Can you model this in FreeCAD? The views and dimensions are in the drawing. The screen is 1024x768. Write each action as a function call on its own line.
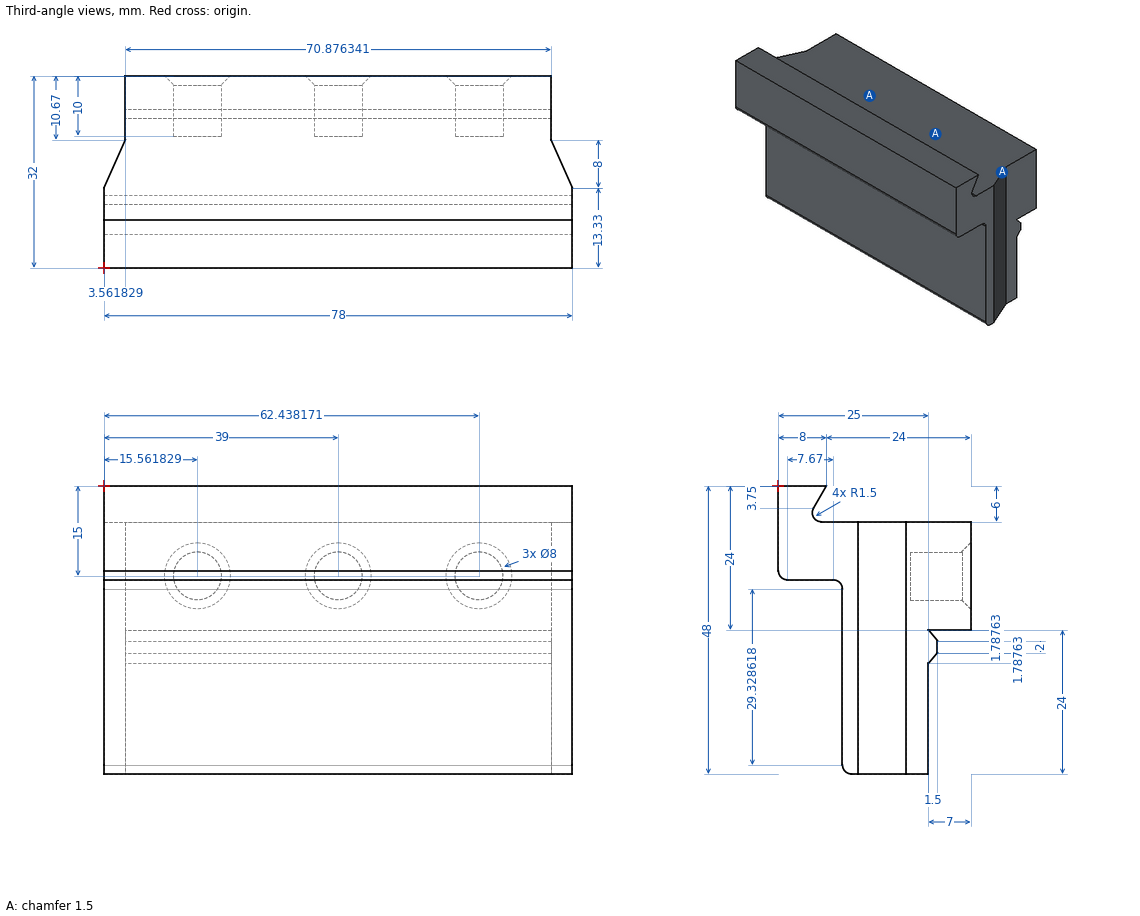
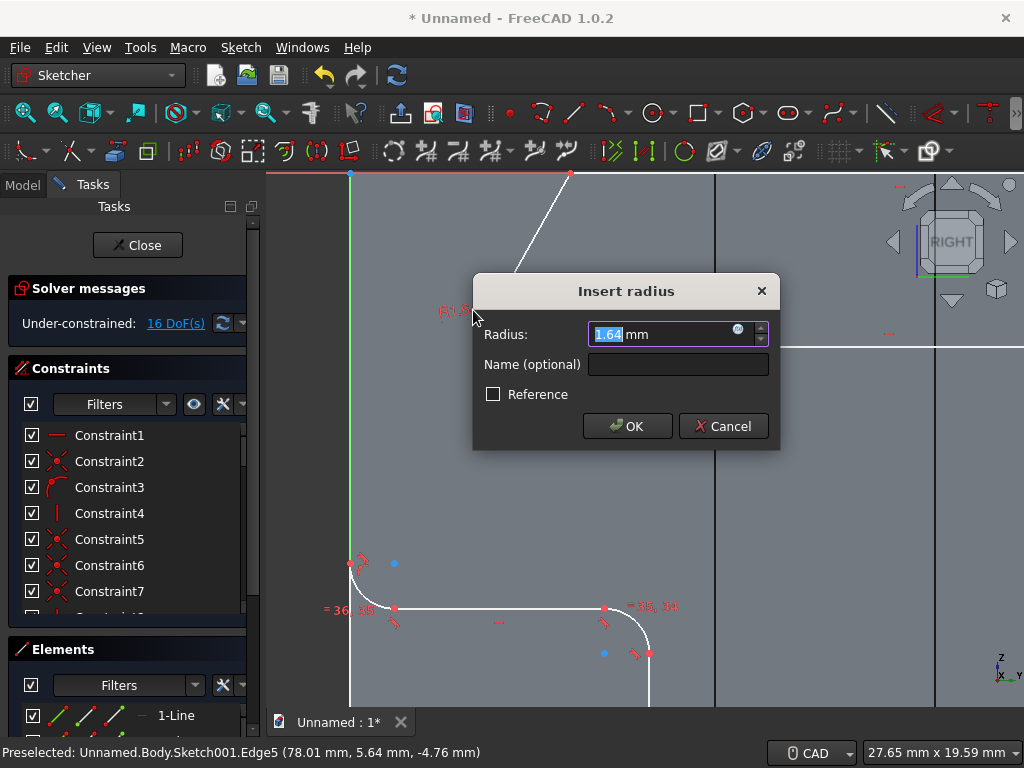
text(1.5)
key(Return)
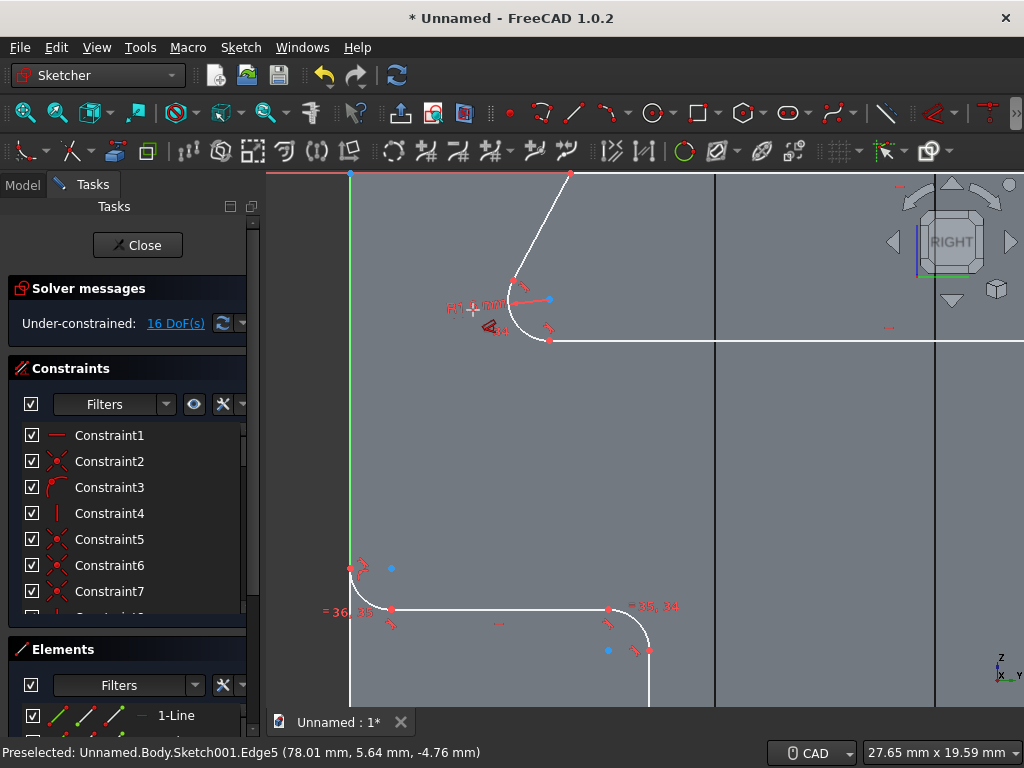
scroll(507, 310, down, 7)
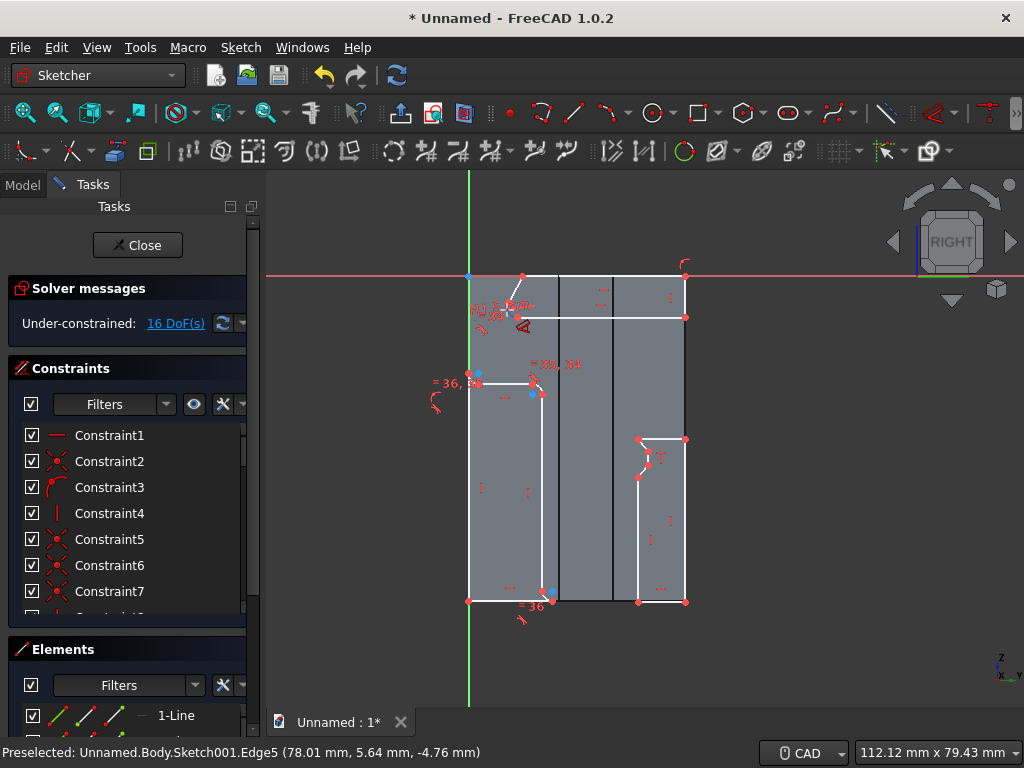
click(685, 305)
click(719, 297)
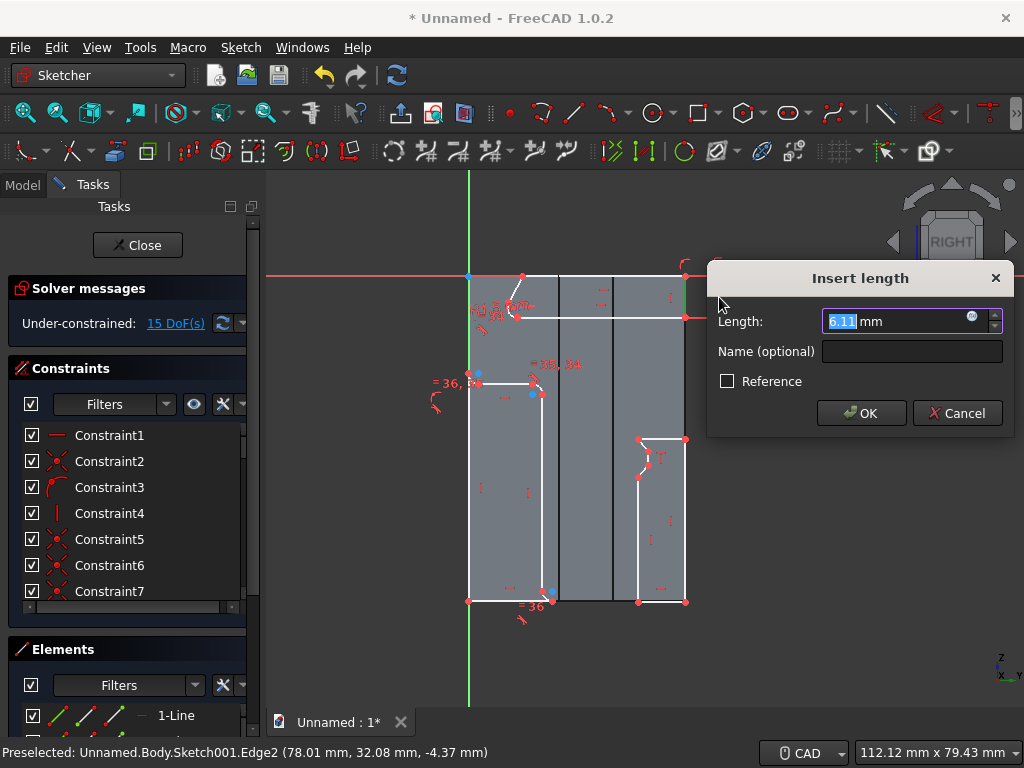
text(6)
key(Return)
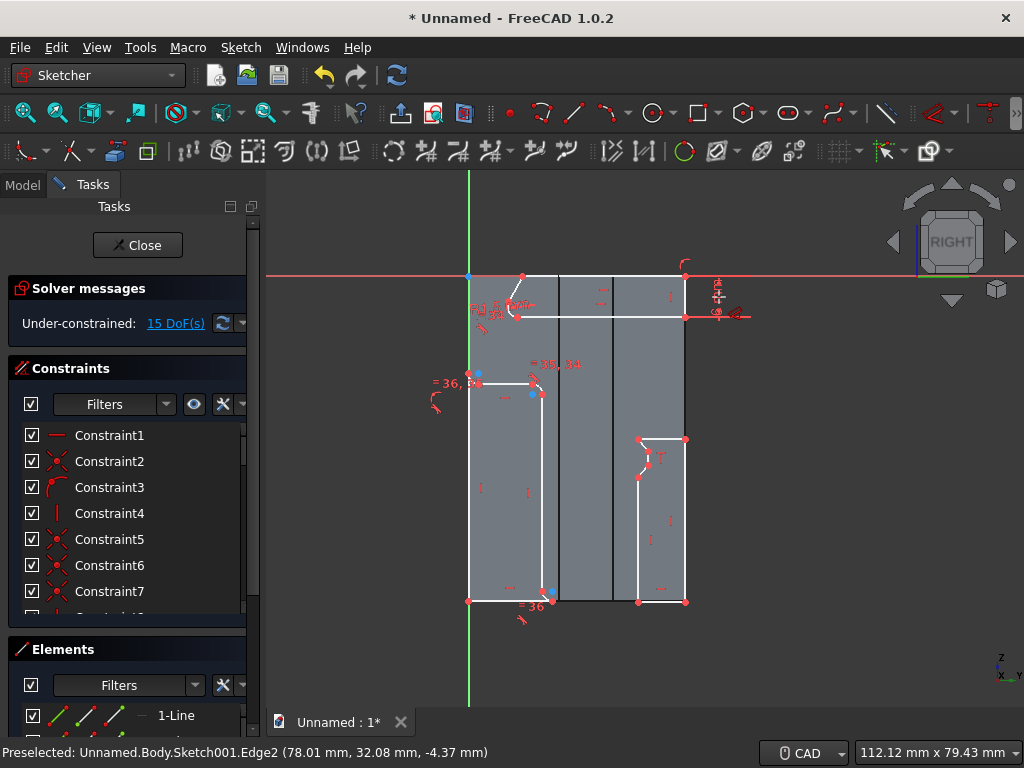
scroll(648, 458, up, 6)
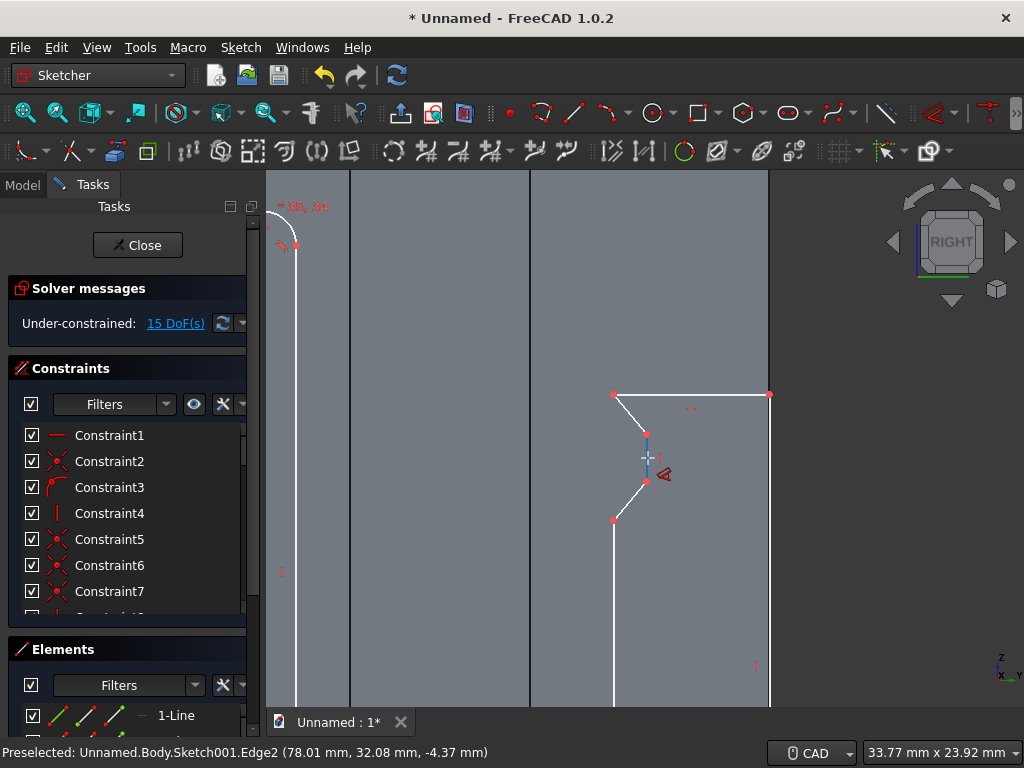
click(647, 458)
click(681, 458)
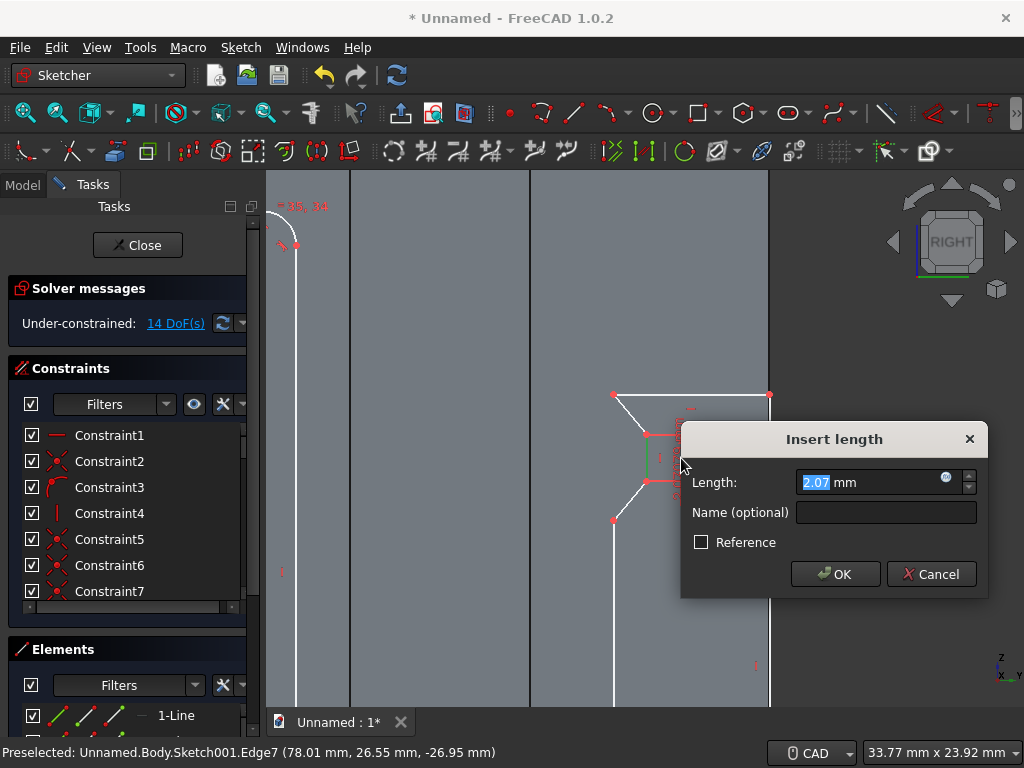
text(2)
key(Return)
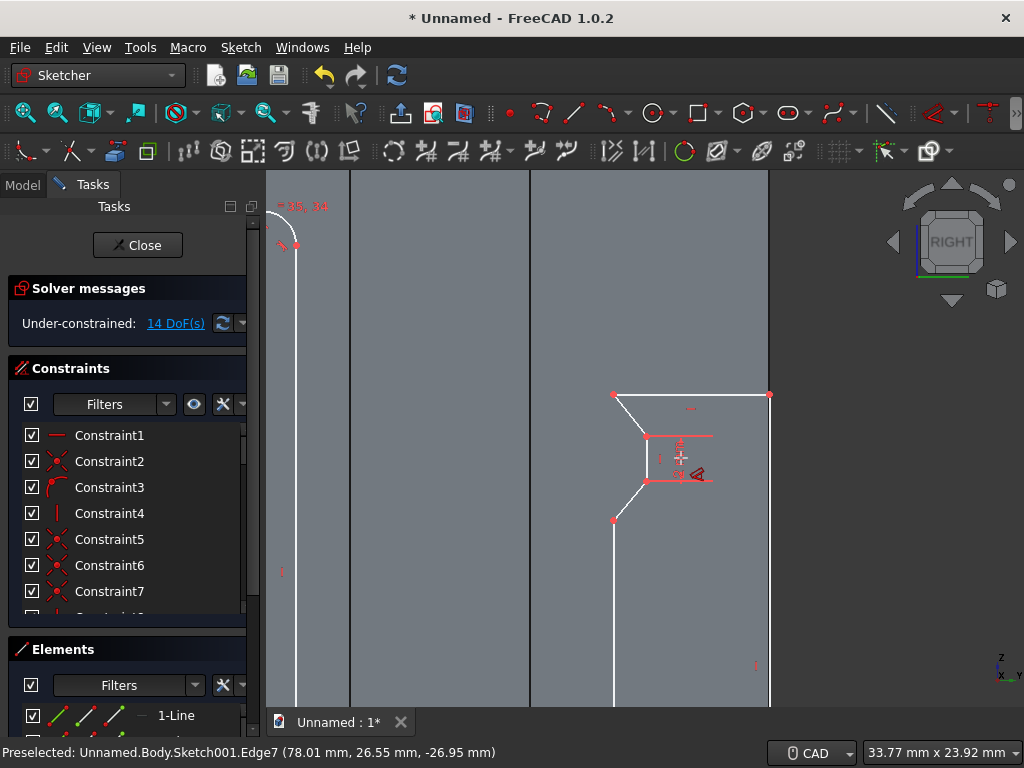
scroll(648, 458, down, 6)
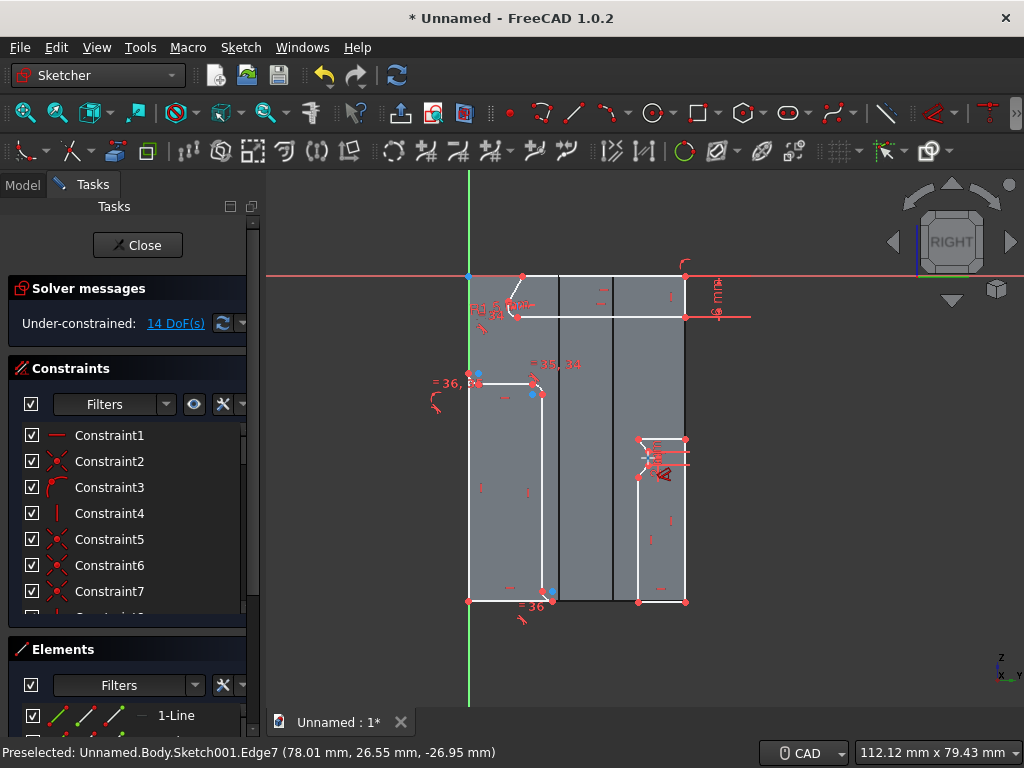
click(652, 602)
click(662, 636)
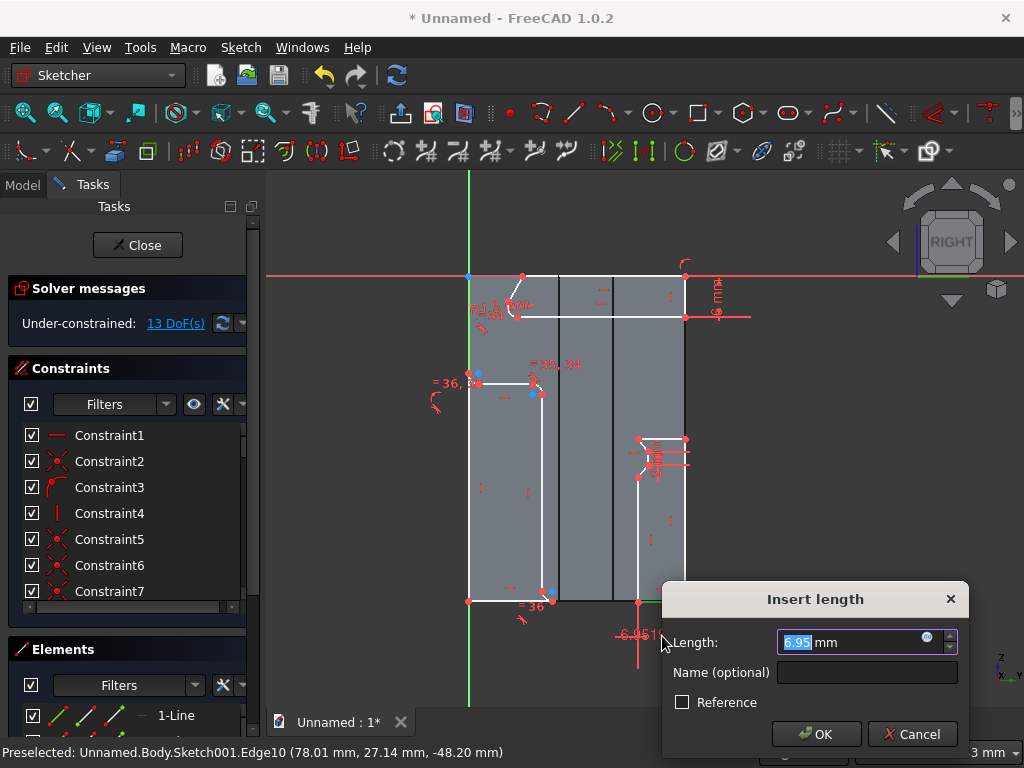
text(7)
key(Return)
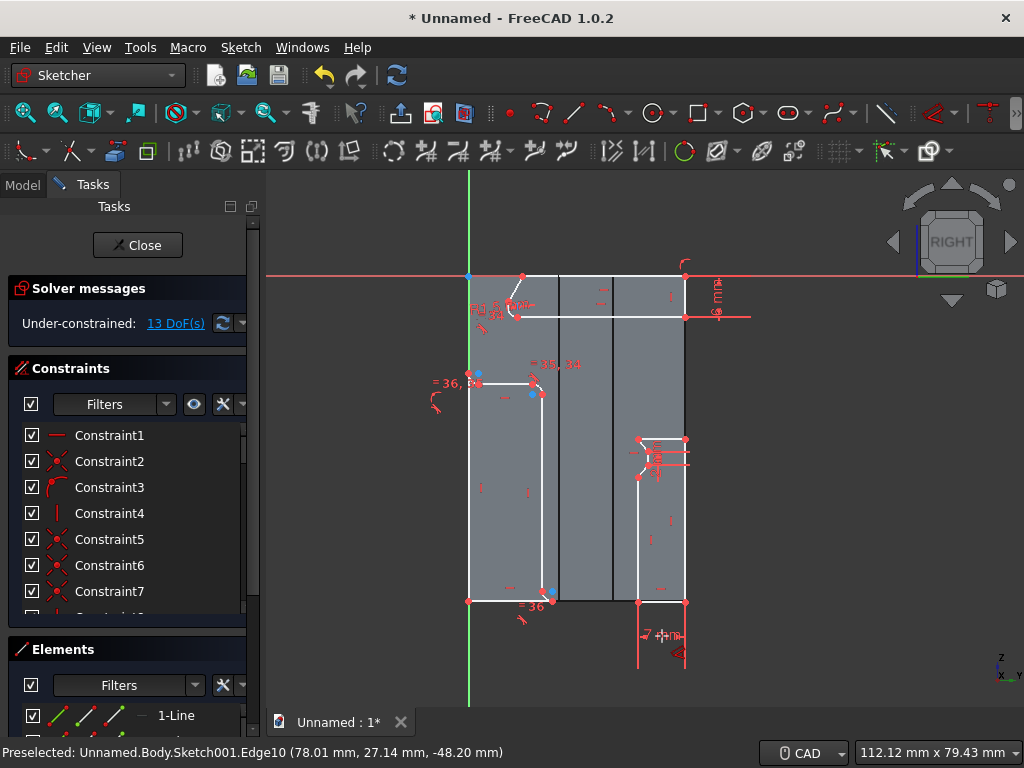
click(671, 439)
click(662, 405)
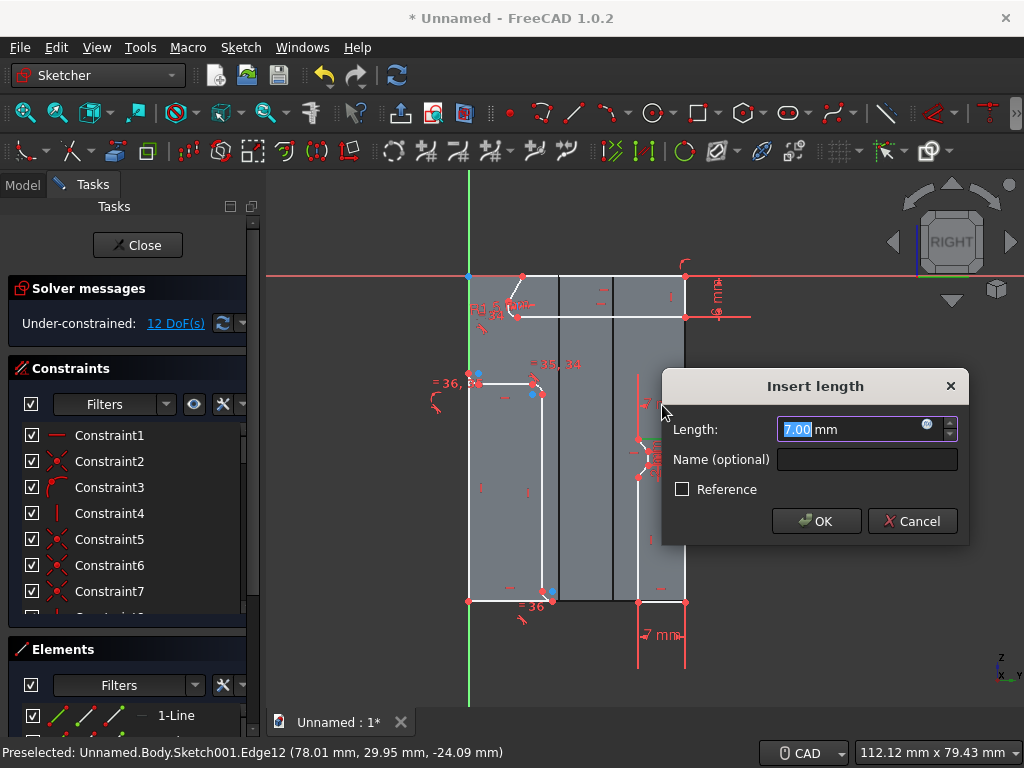
text(7)
key(Return)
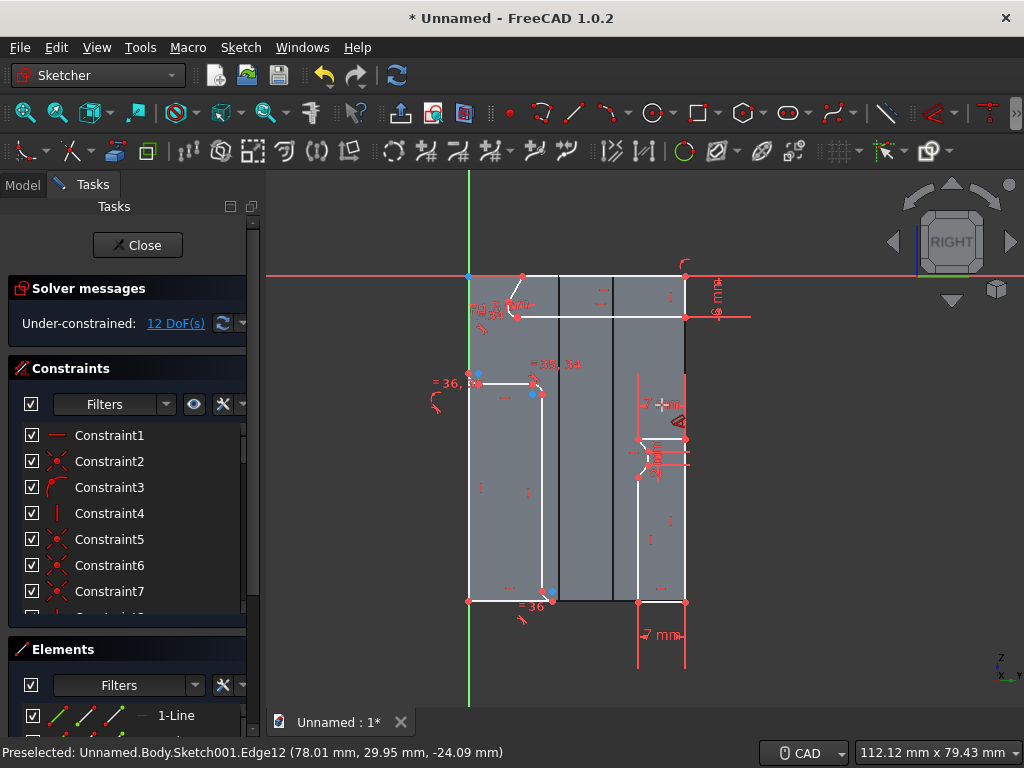
click(637, 276)
click(604, 242)